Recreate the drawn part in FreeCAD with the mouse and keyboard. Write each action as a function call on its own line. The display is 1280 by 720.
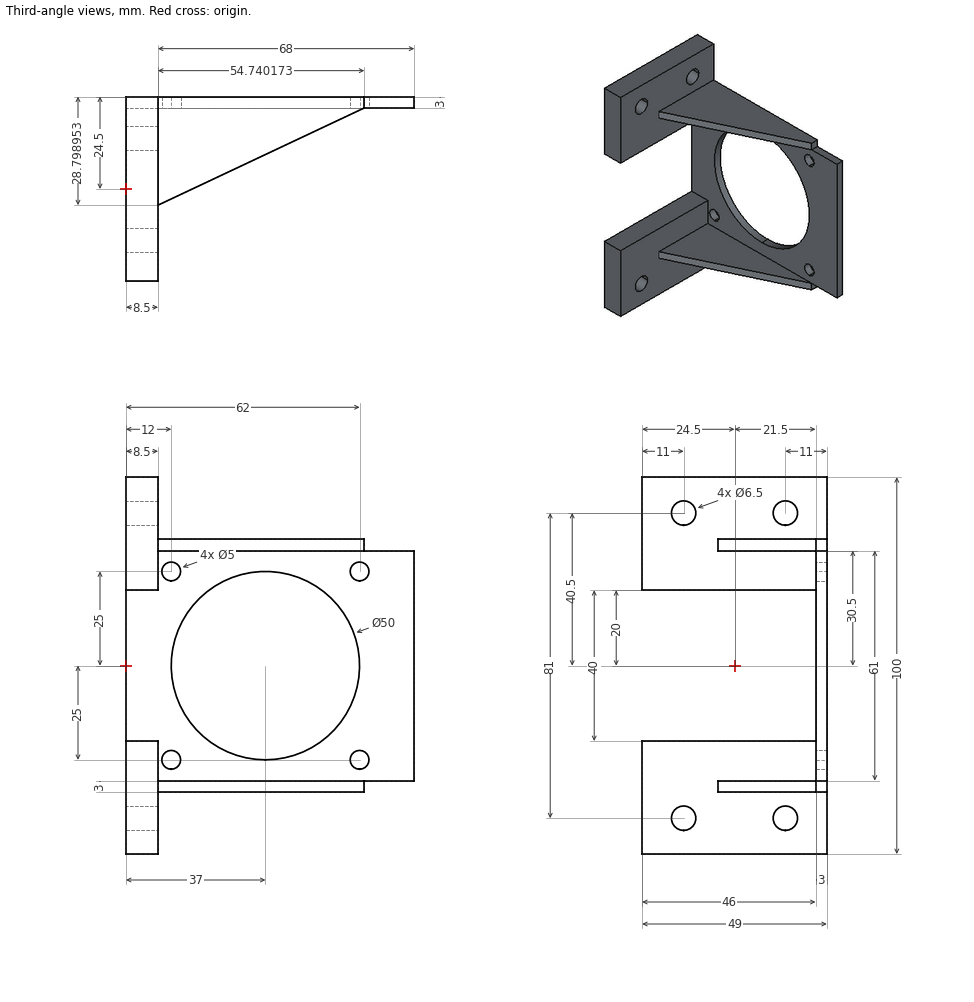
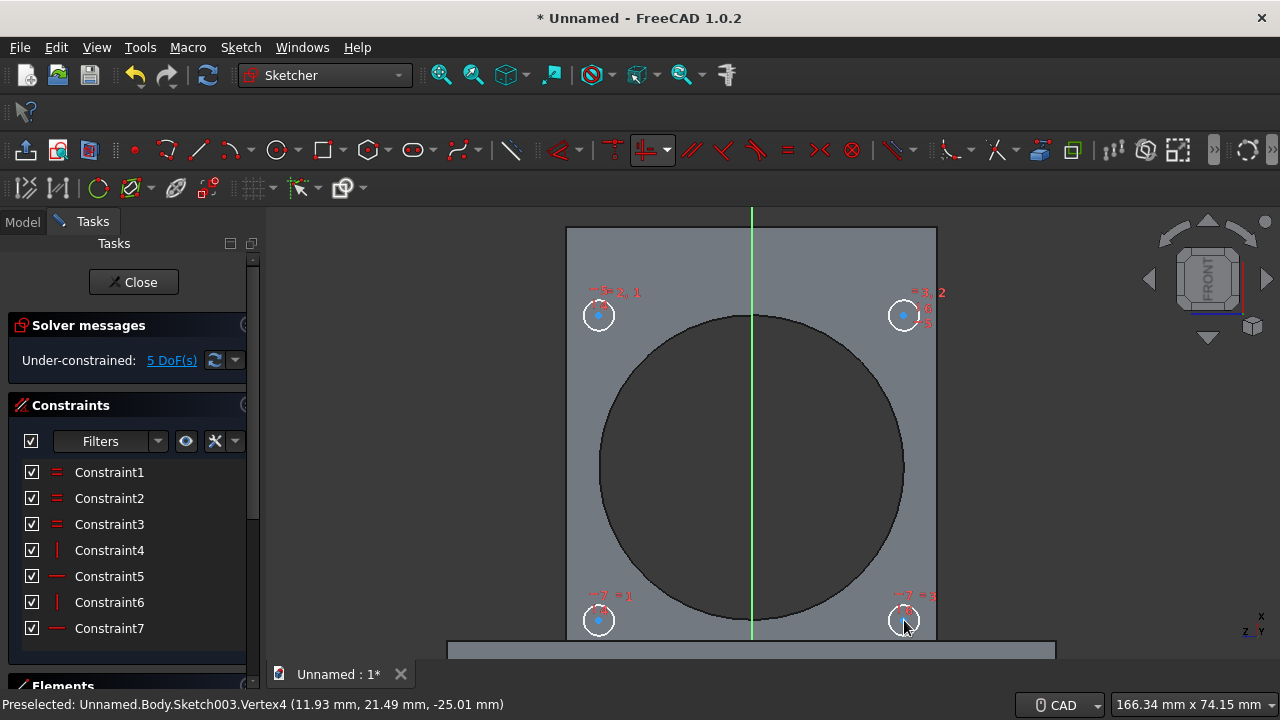
click(558, 150)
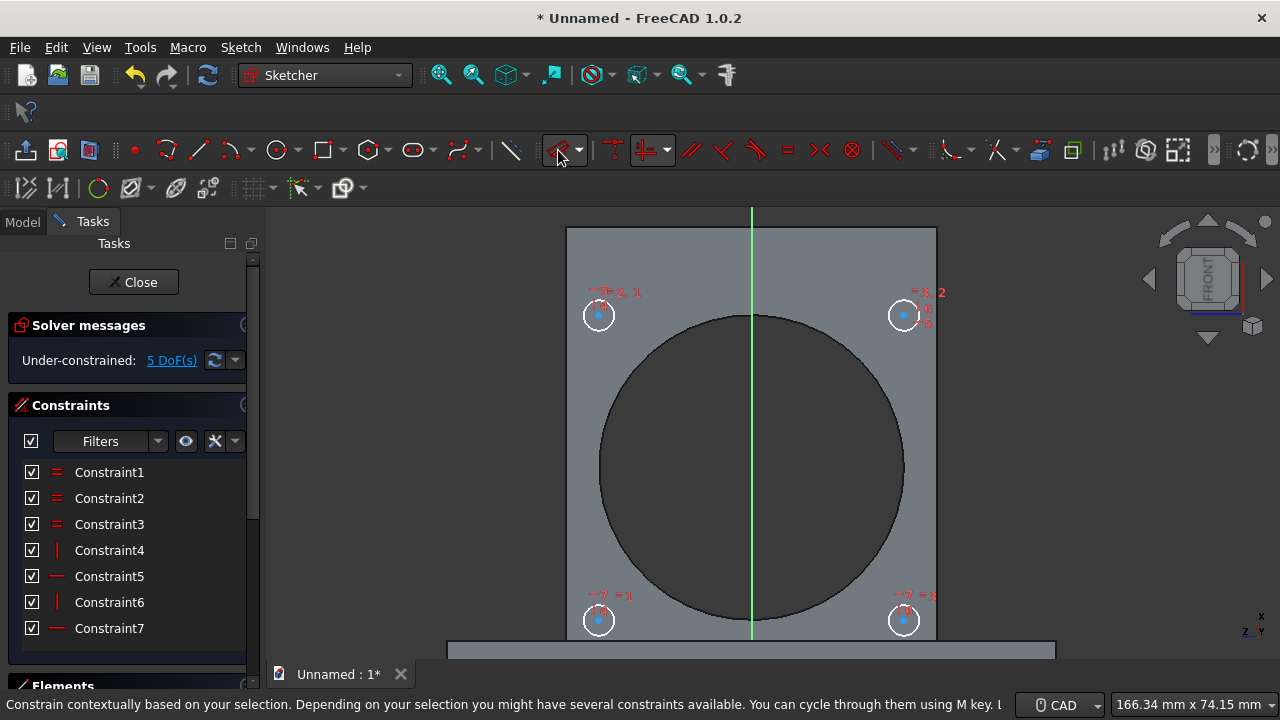
scroll(610, 610, up, 2)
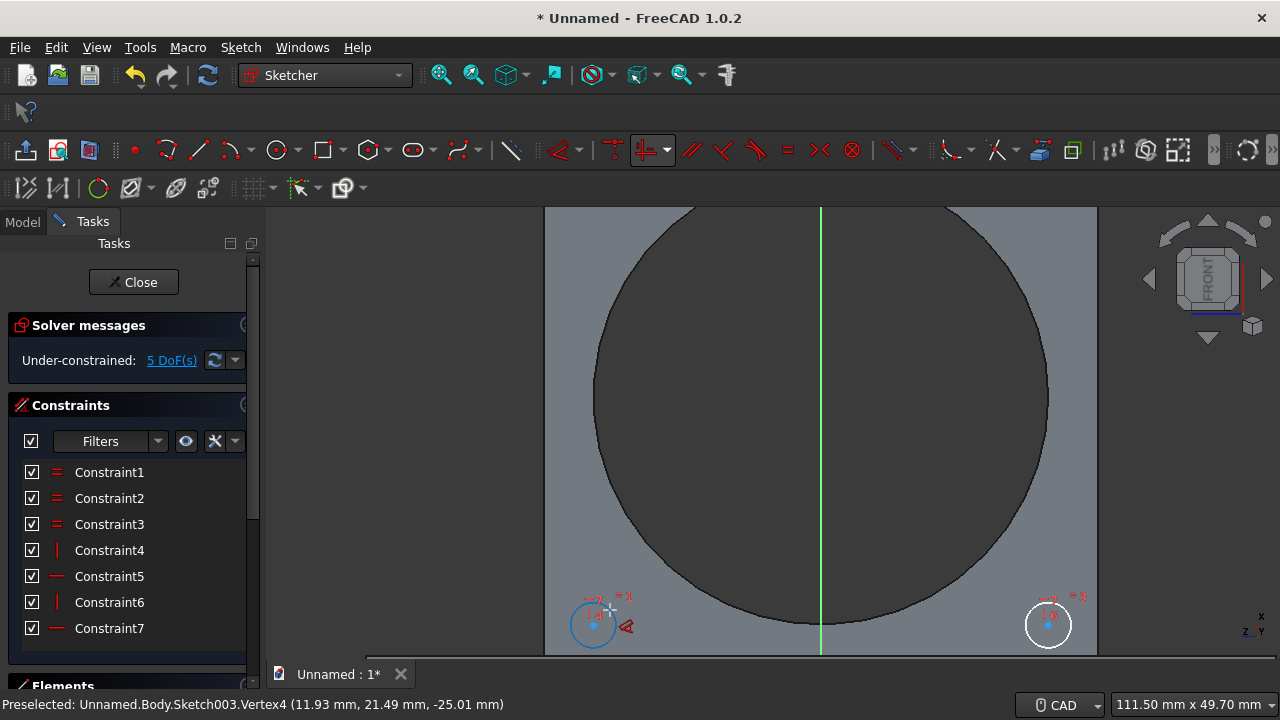
click(609, 609)
click(631, 586)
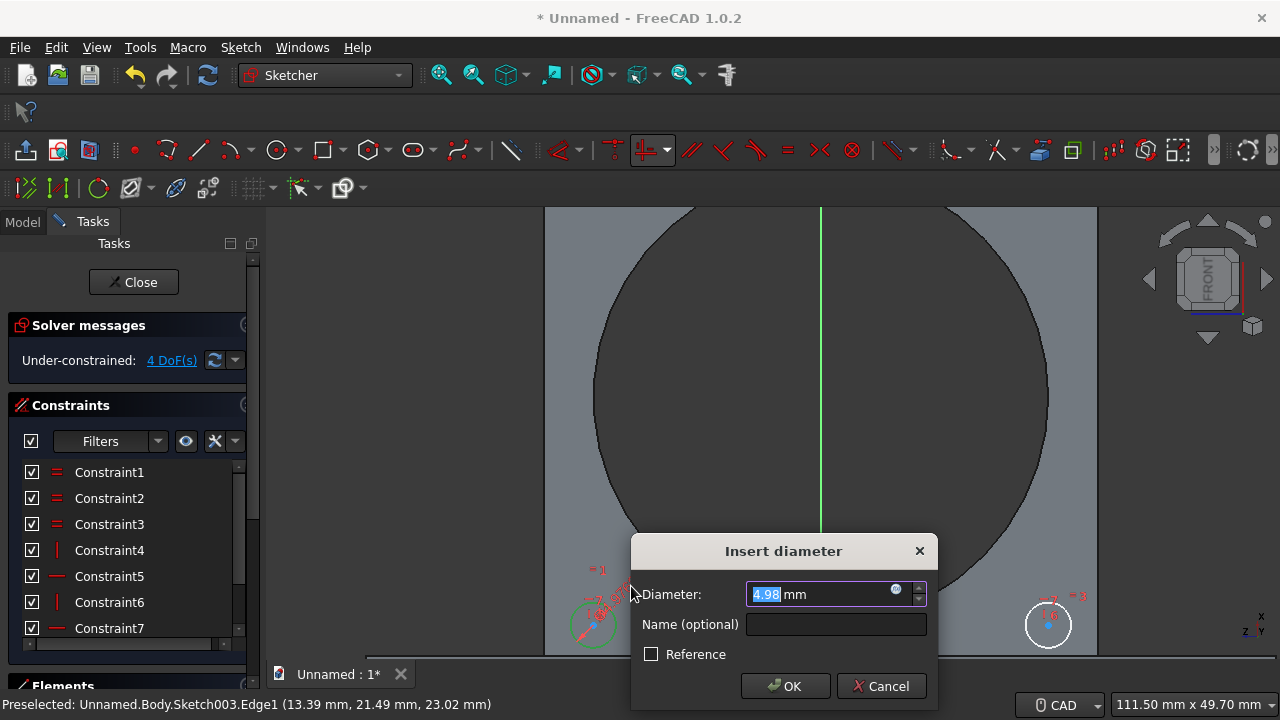
text(5)
key(Return)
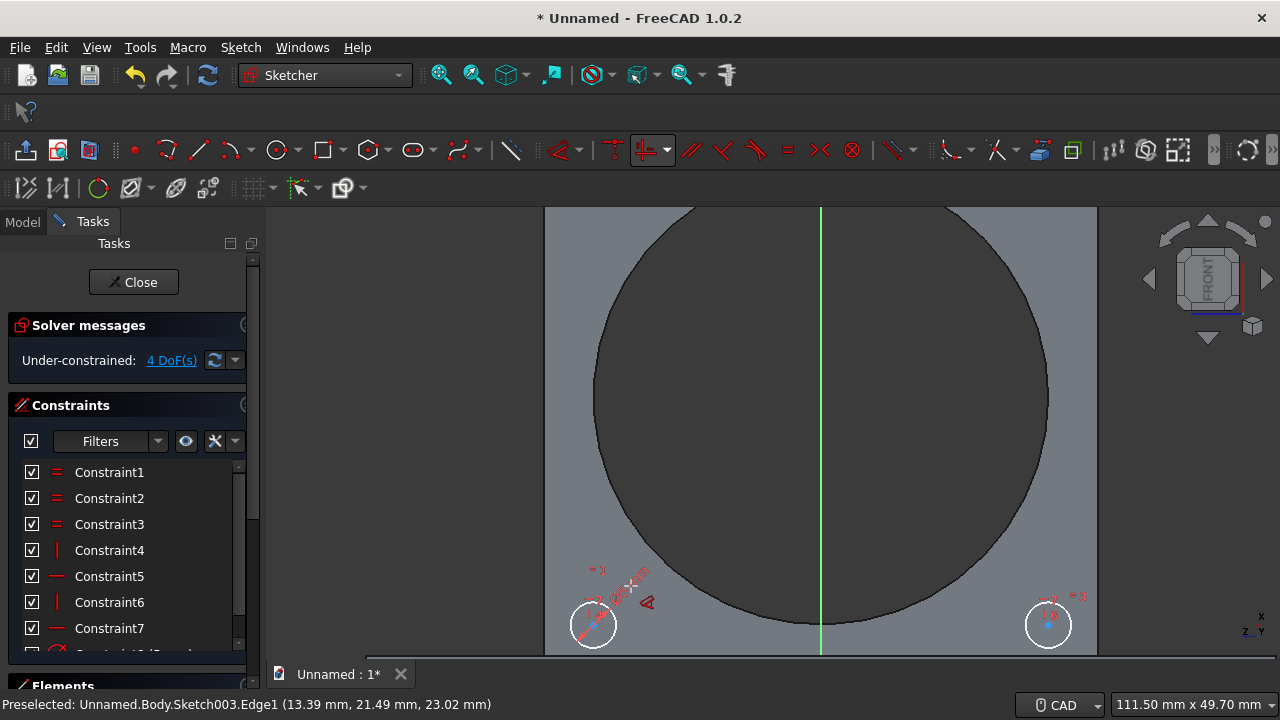
click(593, 625)
click(707, 591)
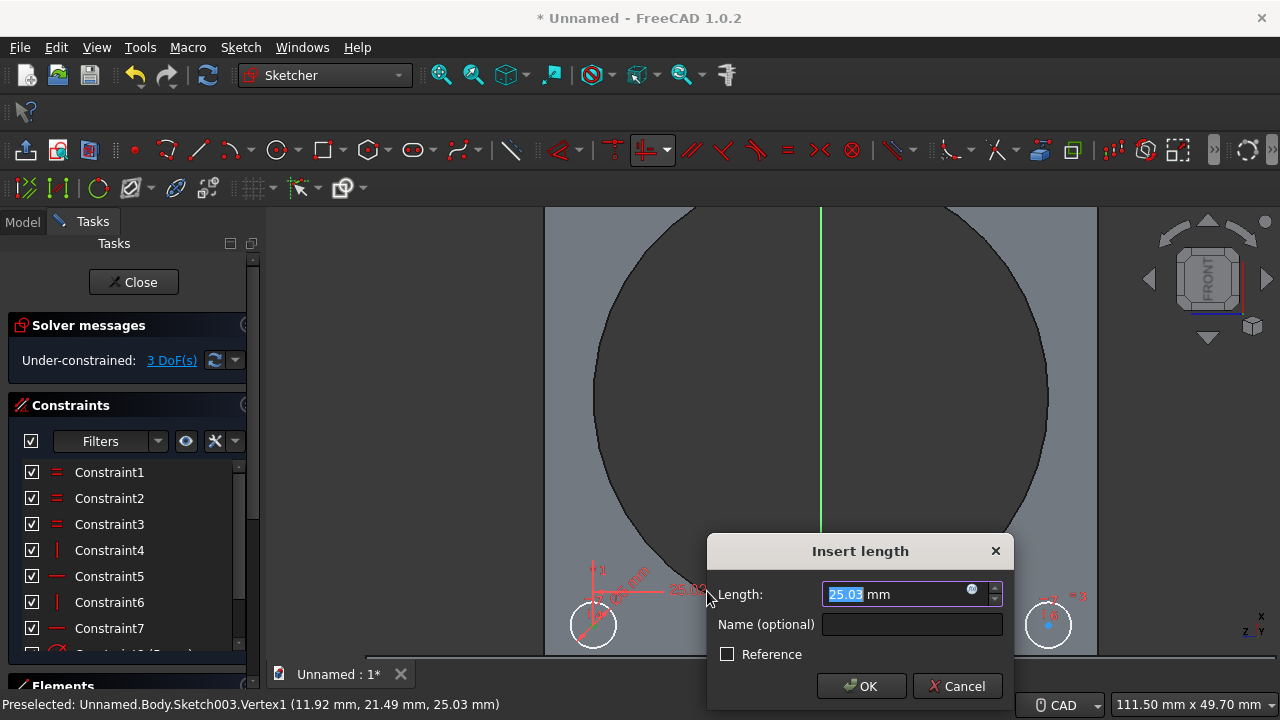
text(25)
key(Return)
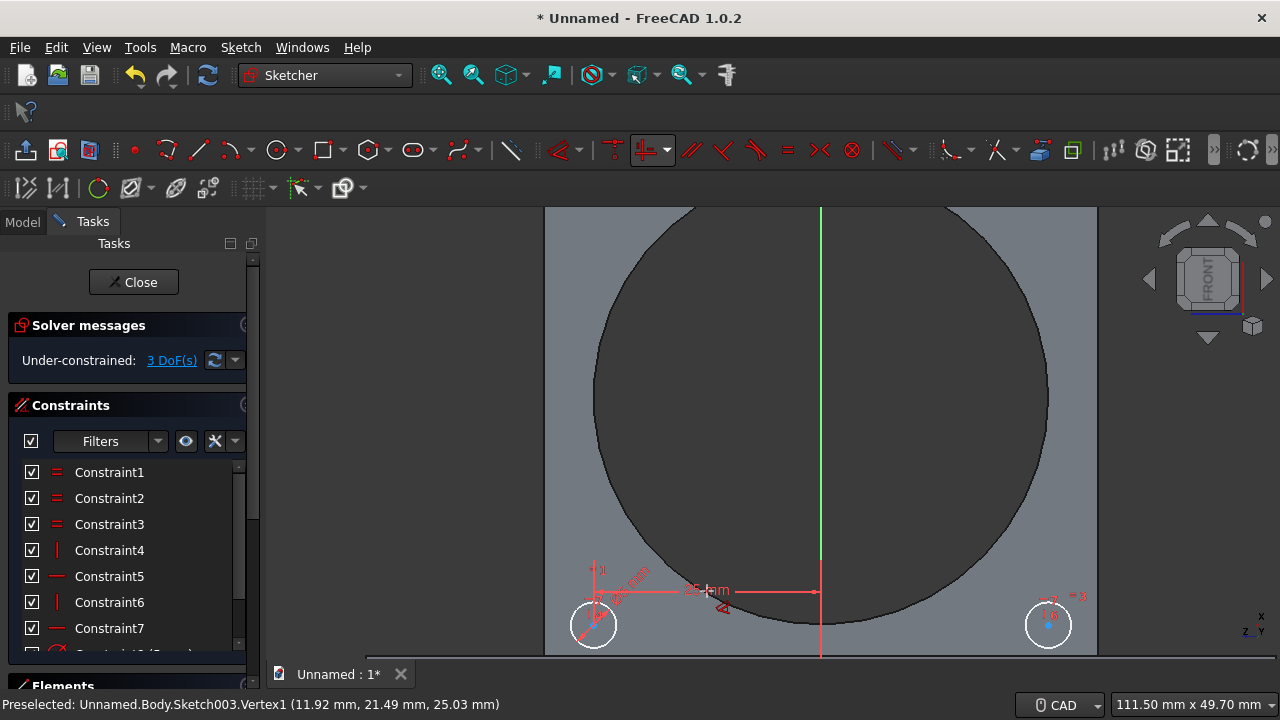
click(594, 625)
click(855, 628)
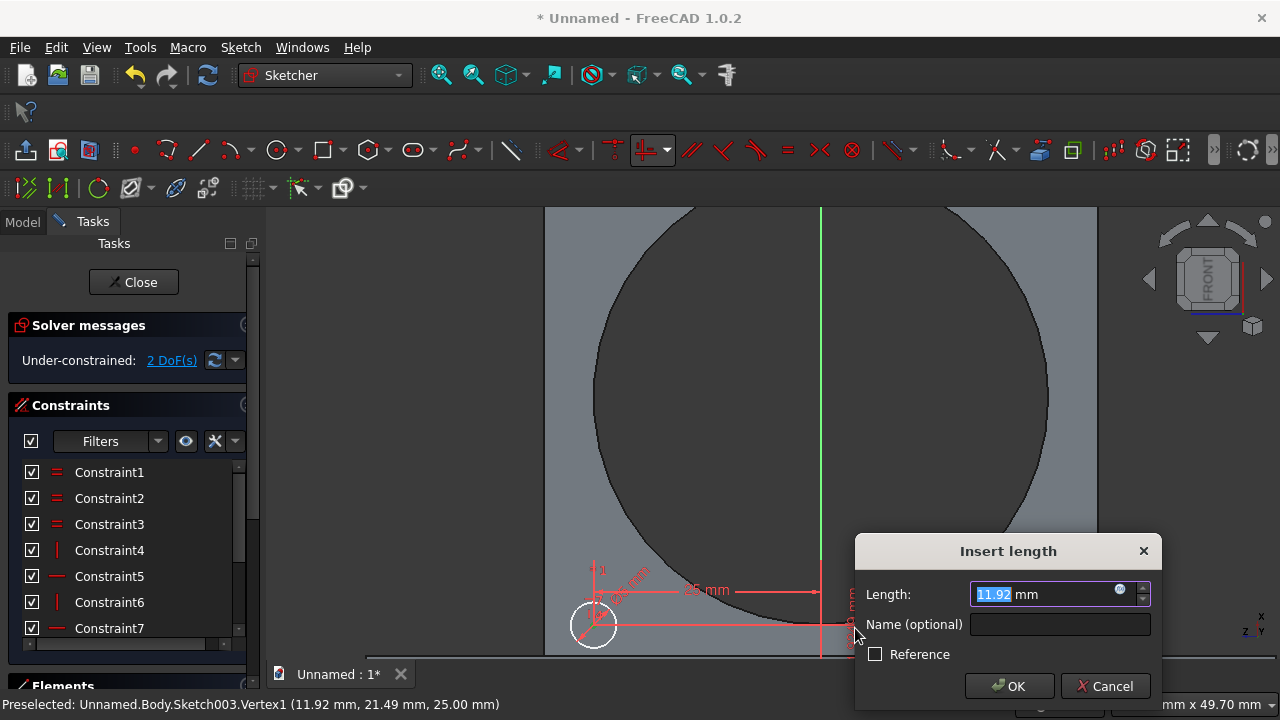
text(12)
key(Return)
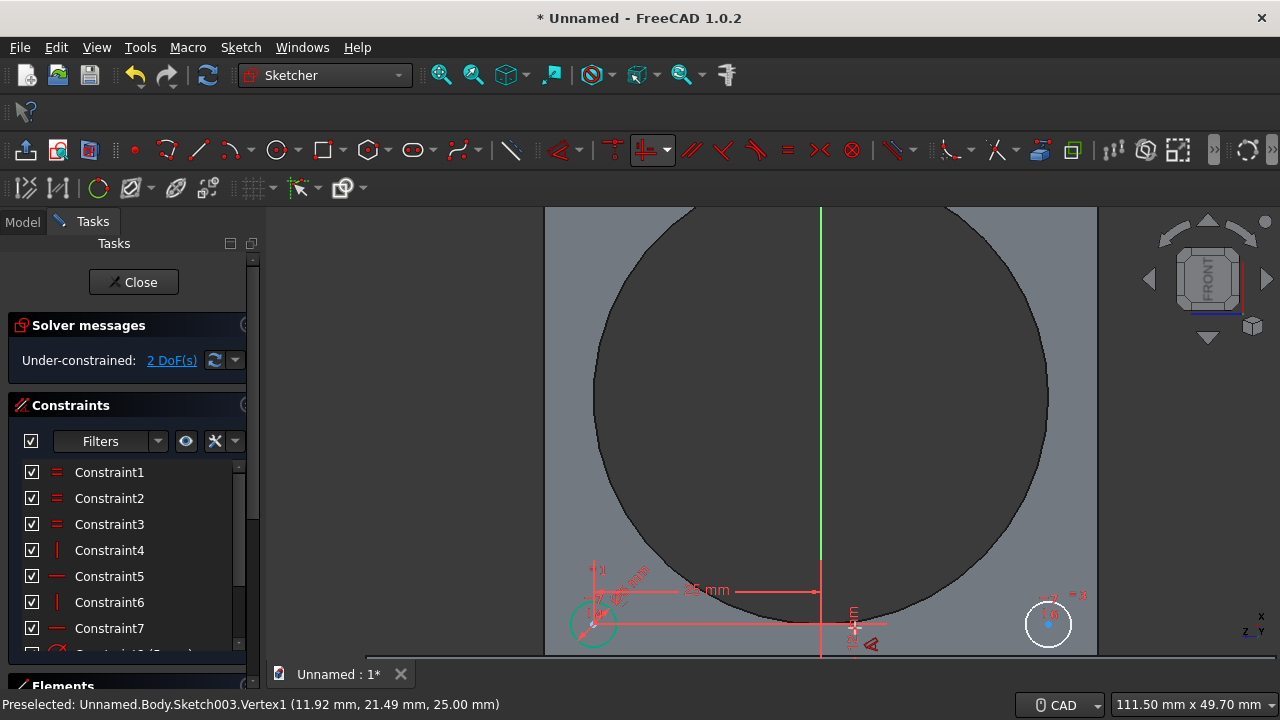
scroll(609, 427, down, 4)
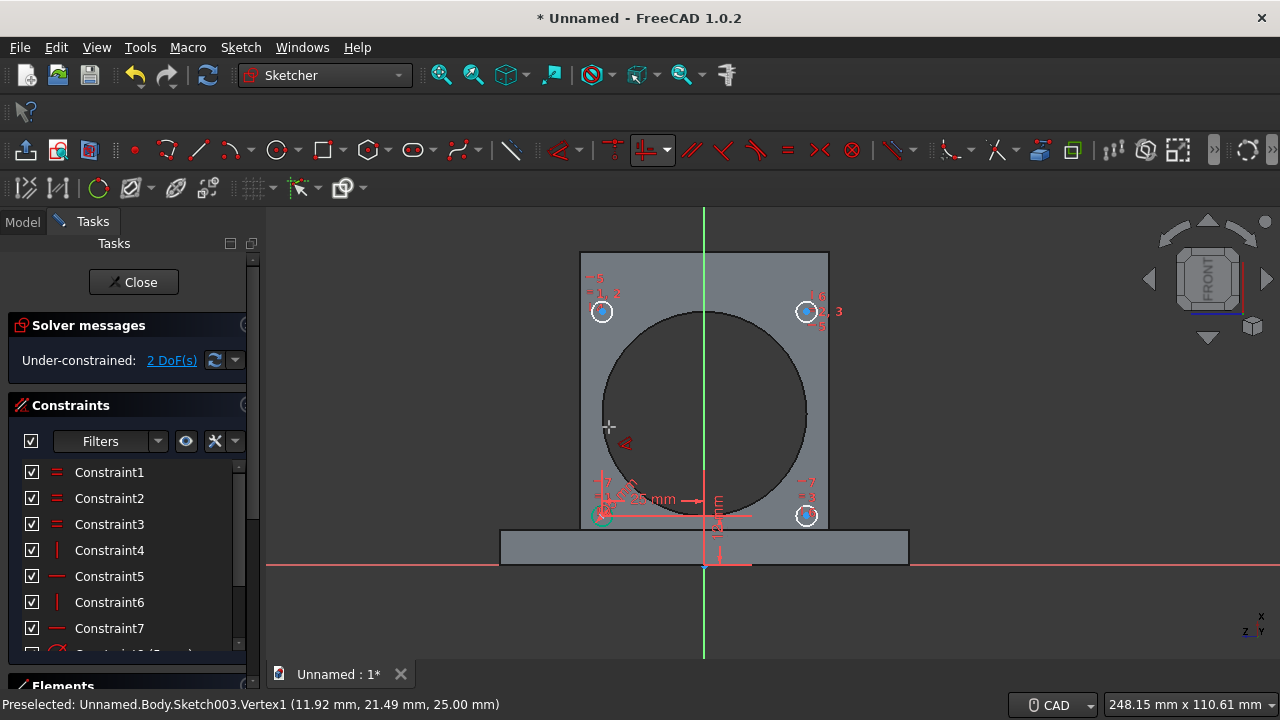
click(602, 312)
click(568, 438)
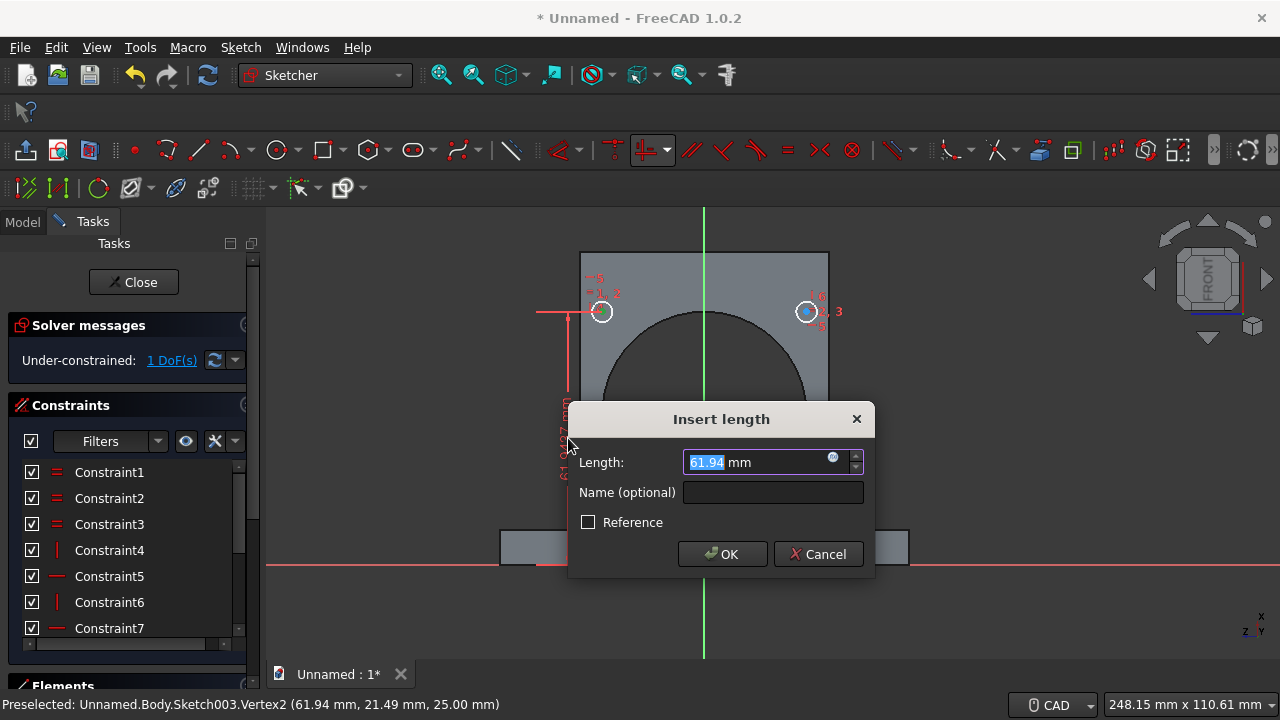
text(62)
key(Return)